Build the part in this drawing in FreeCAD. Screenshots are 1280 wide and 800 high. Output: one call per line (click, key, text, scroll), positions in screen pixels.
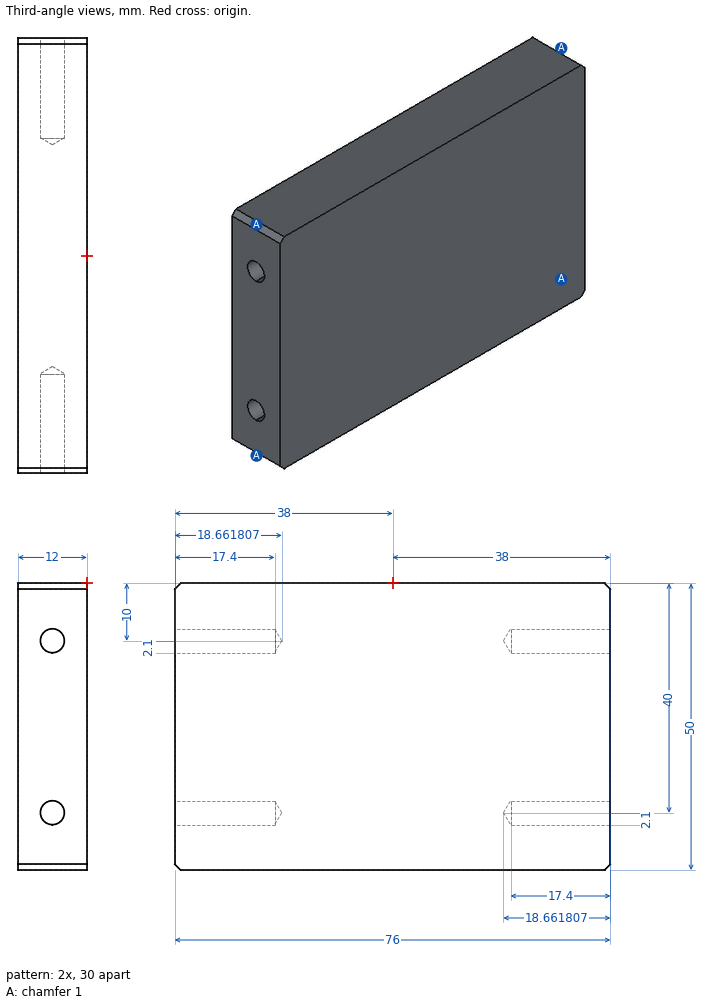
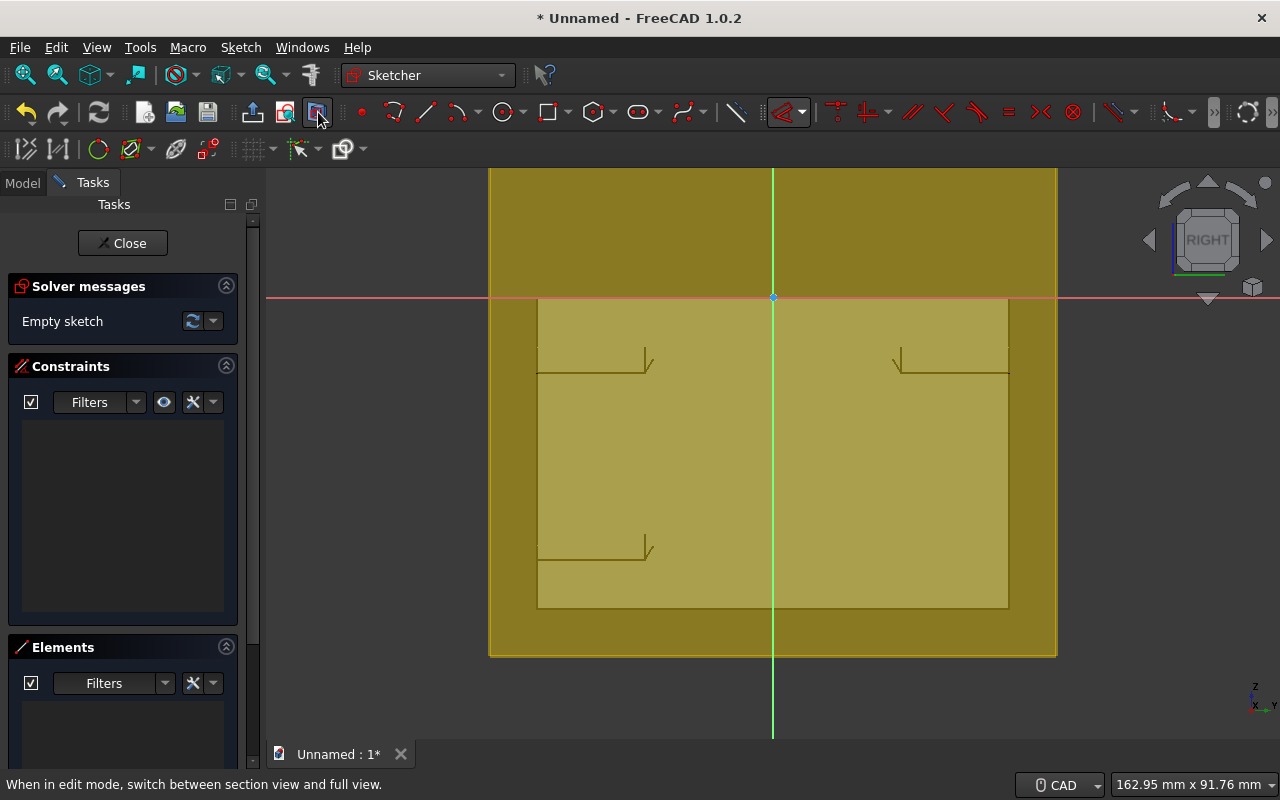
scroll(1115, 379, up, 2)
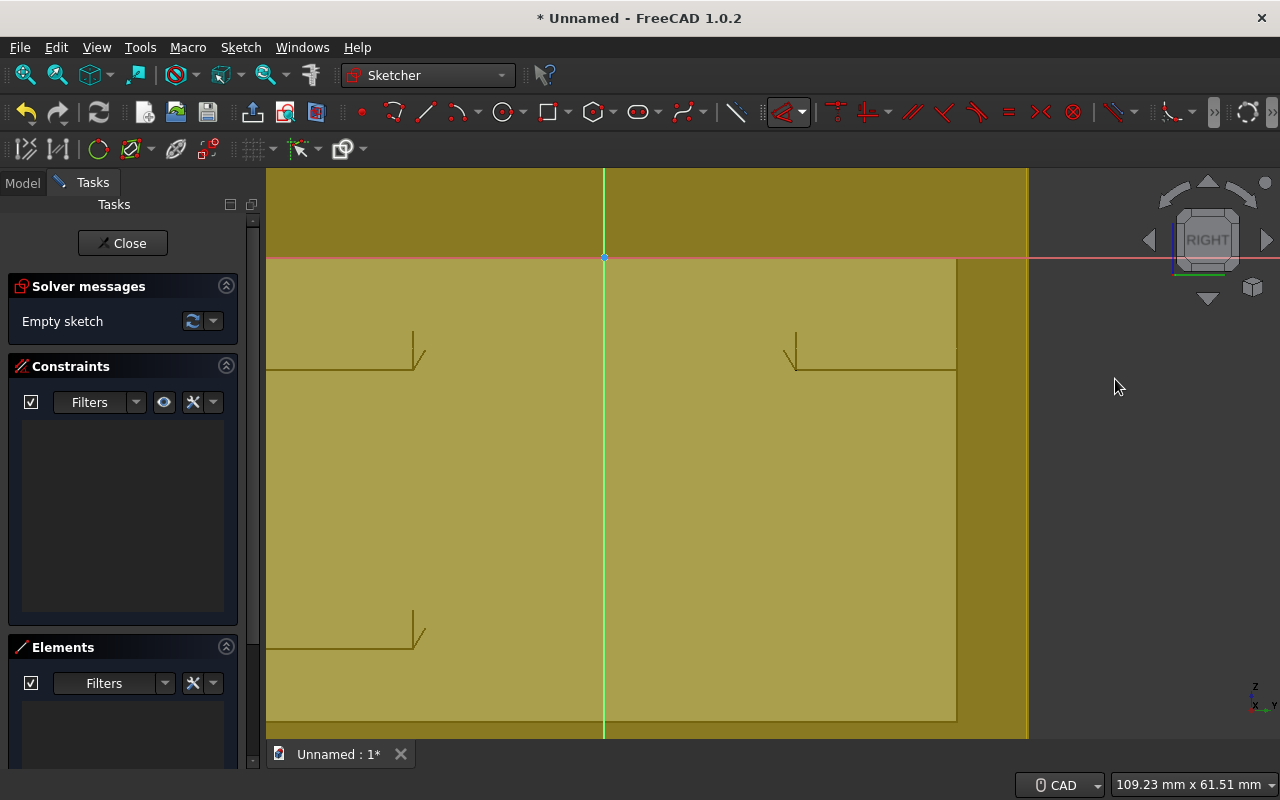
click(394, 112)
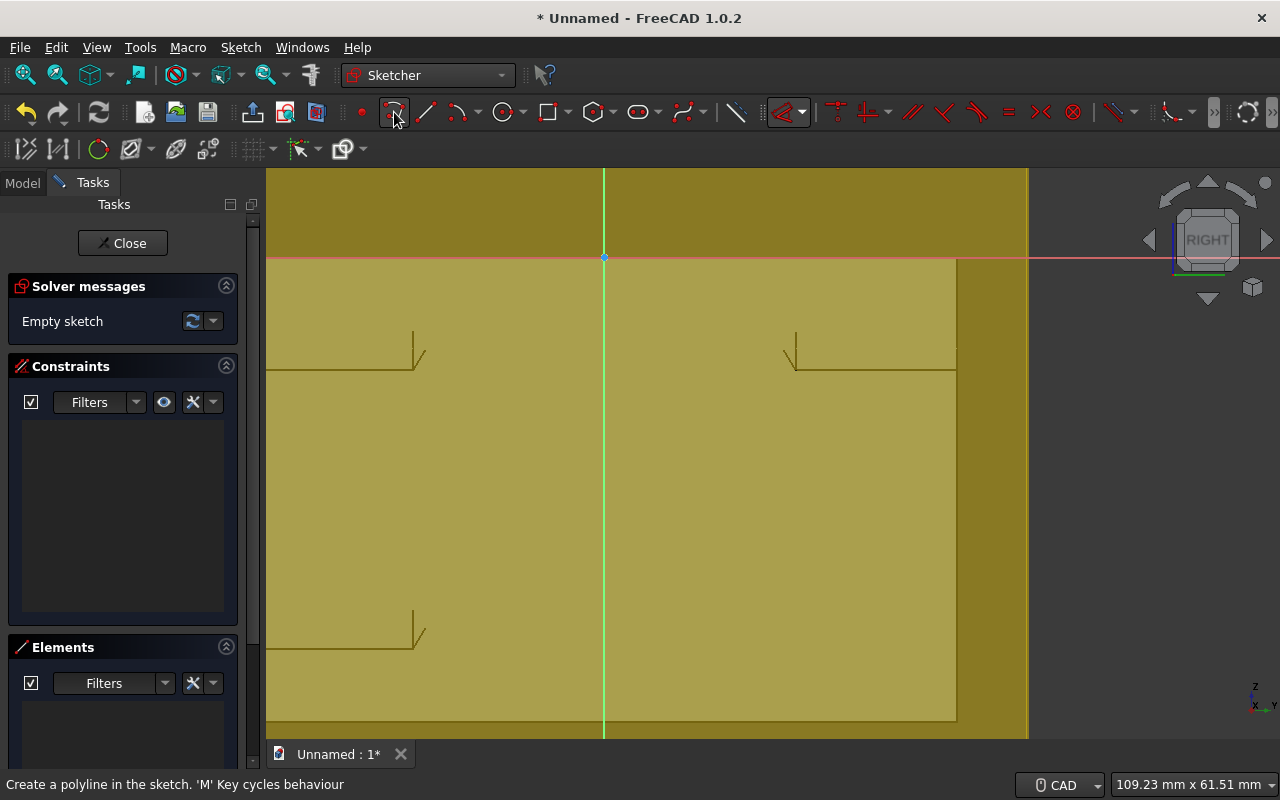
click(784, 629)
click(796, 649)
click(957, 649)
click(957, 629)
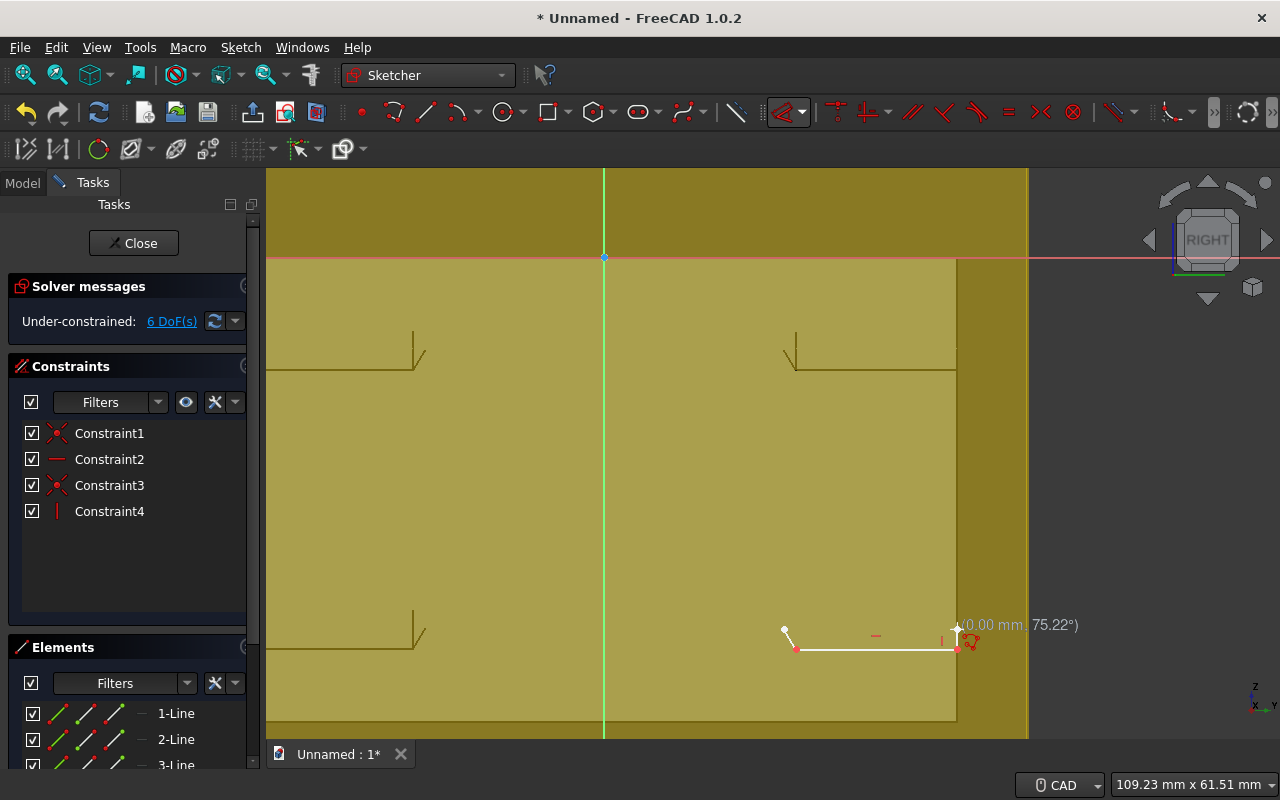
scroll(784, 629, up, 2)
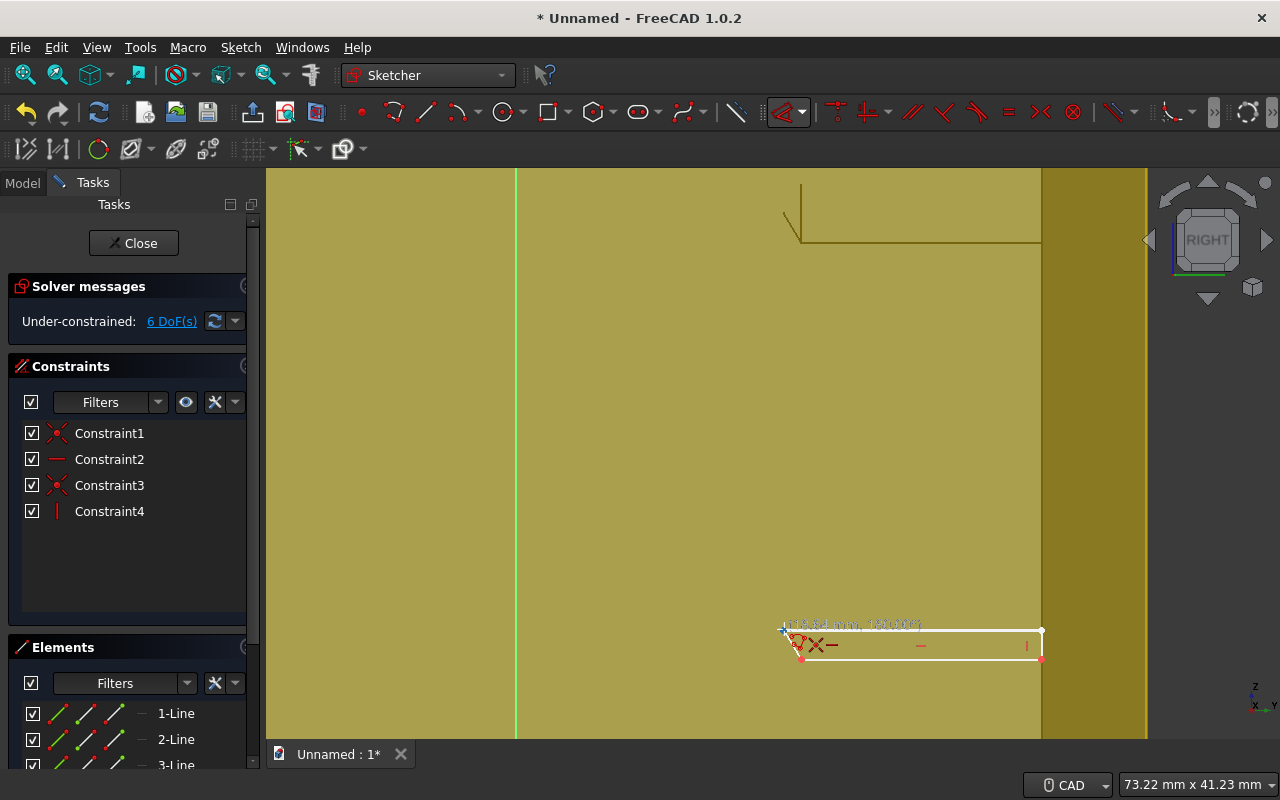
click(784, 630)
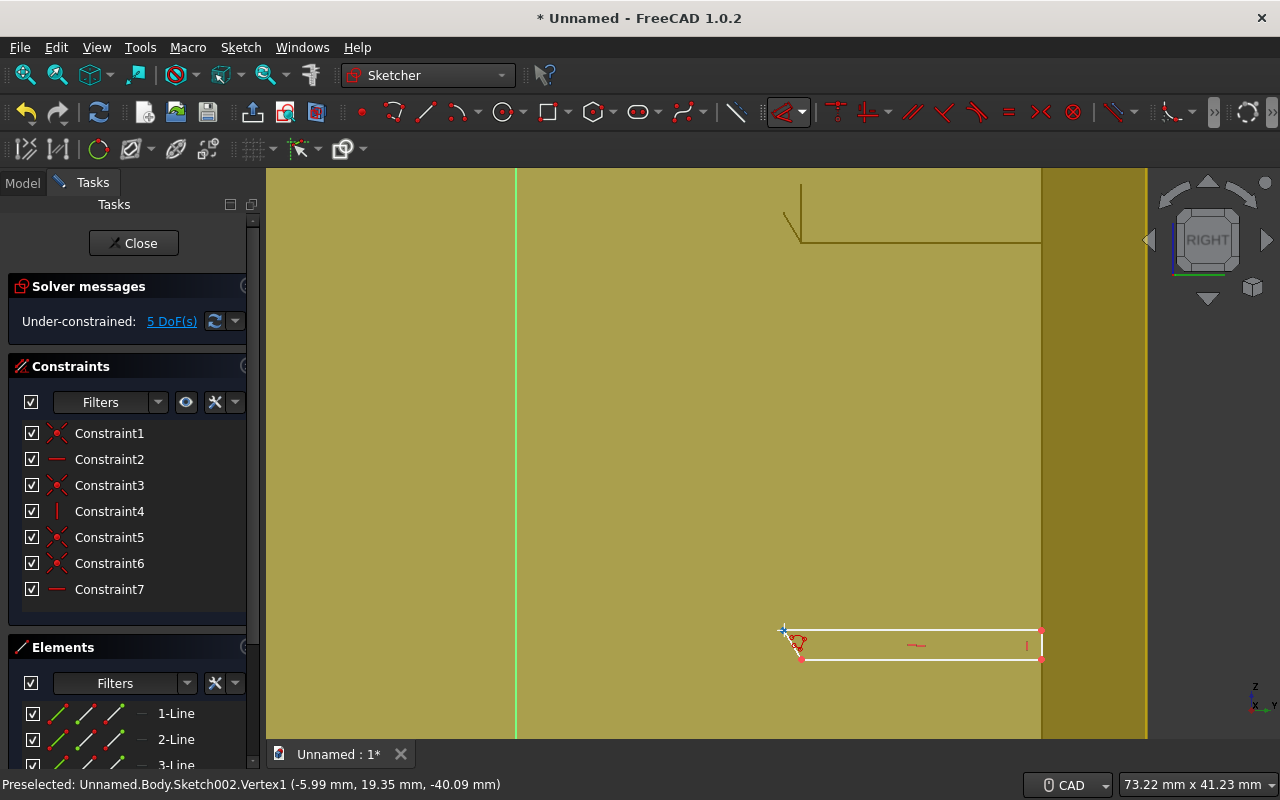
click(426, 112)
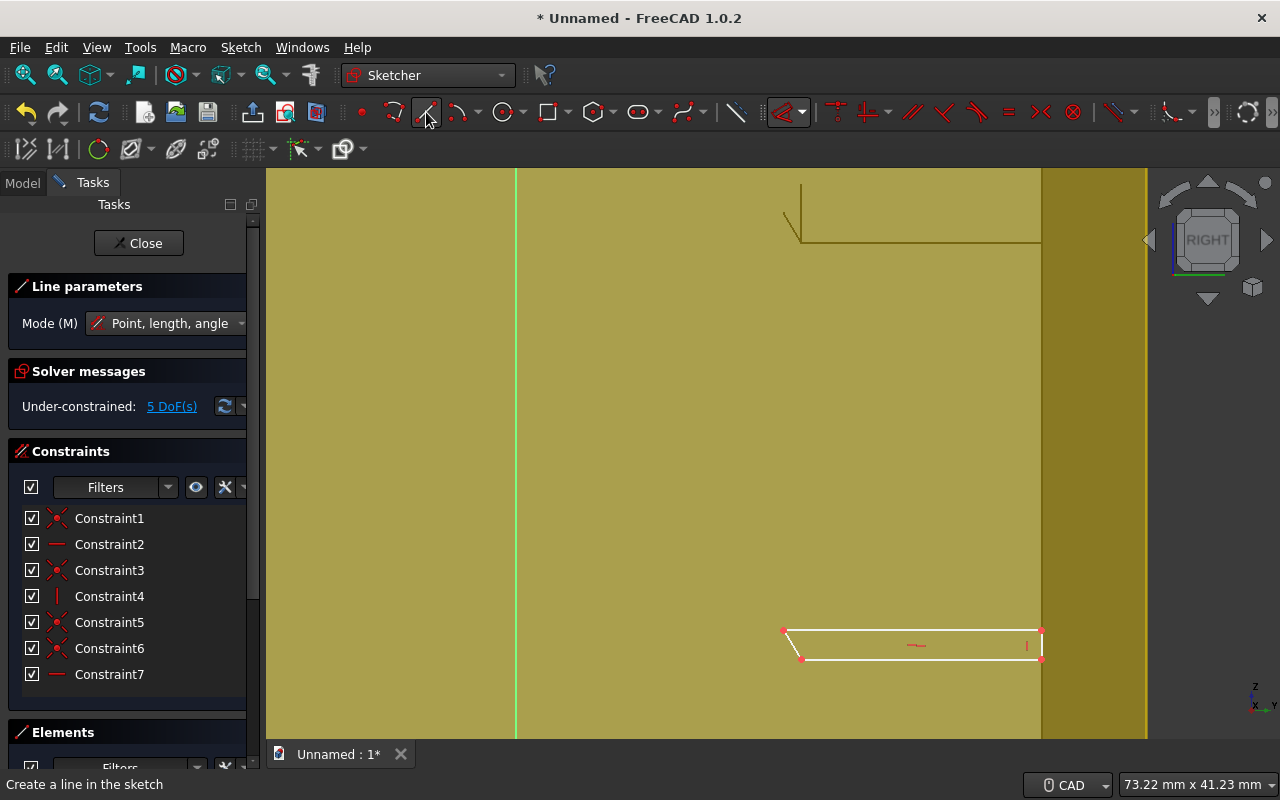
click(1068, 629)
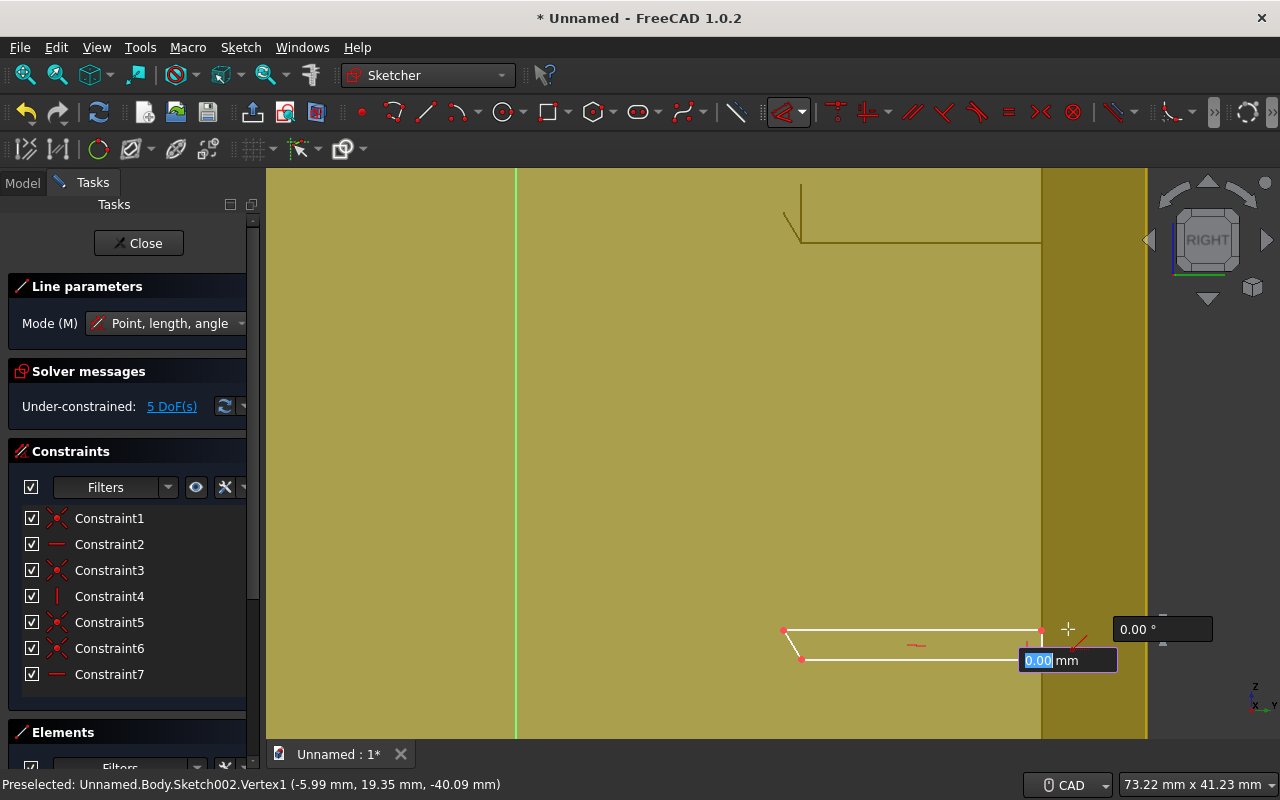
scroll(448, 630, down, 2)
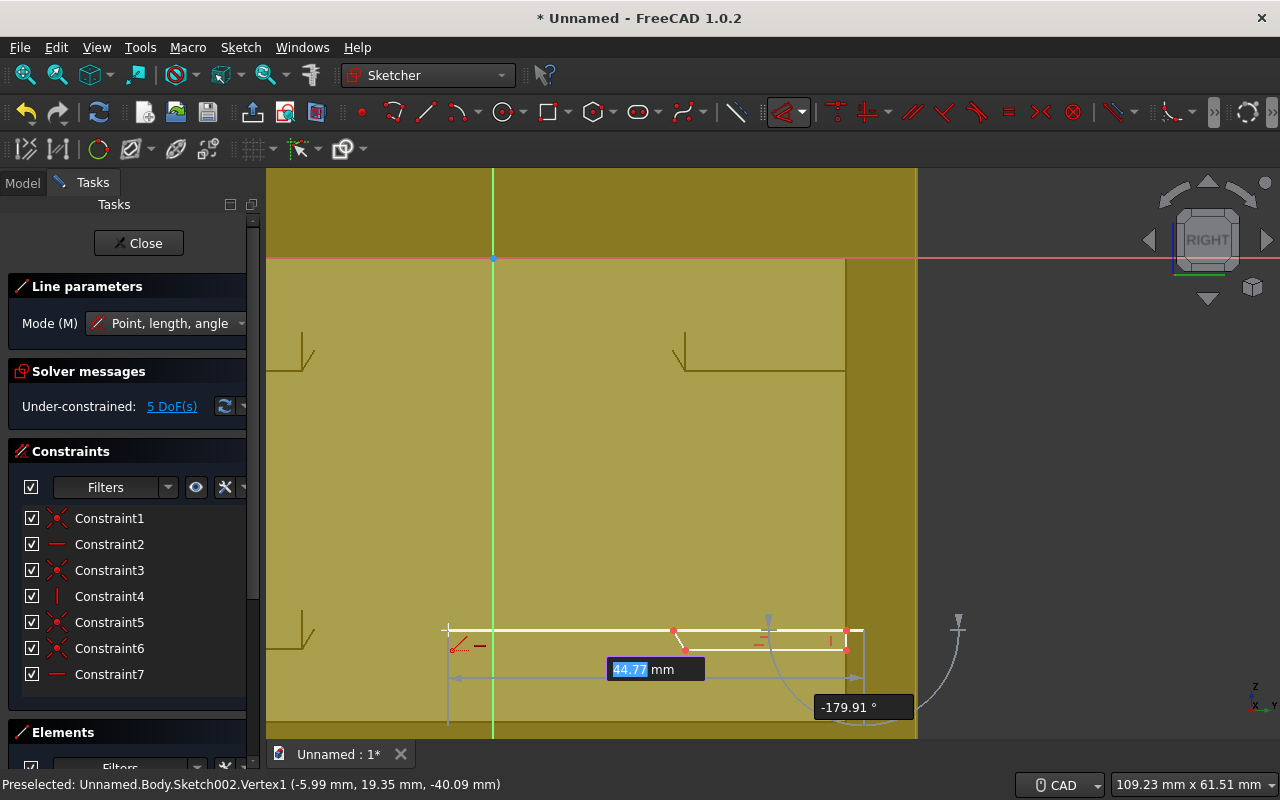
click(916, 630)
key(Escape)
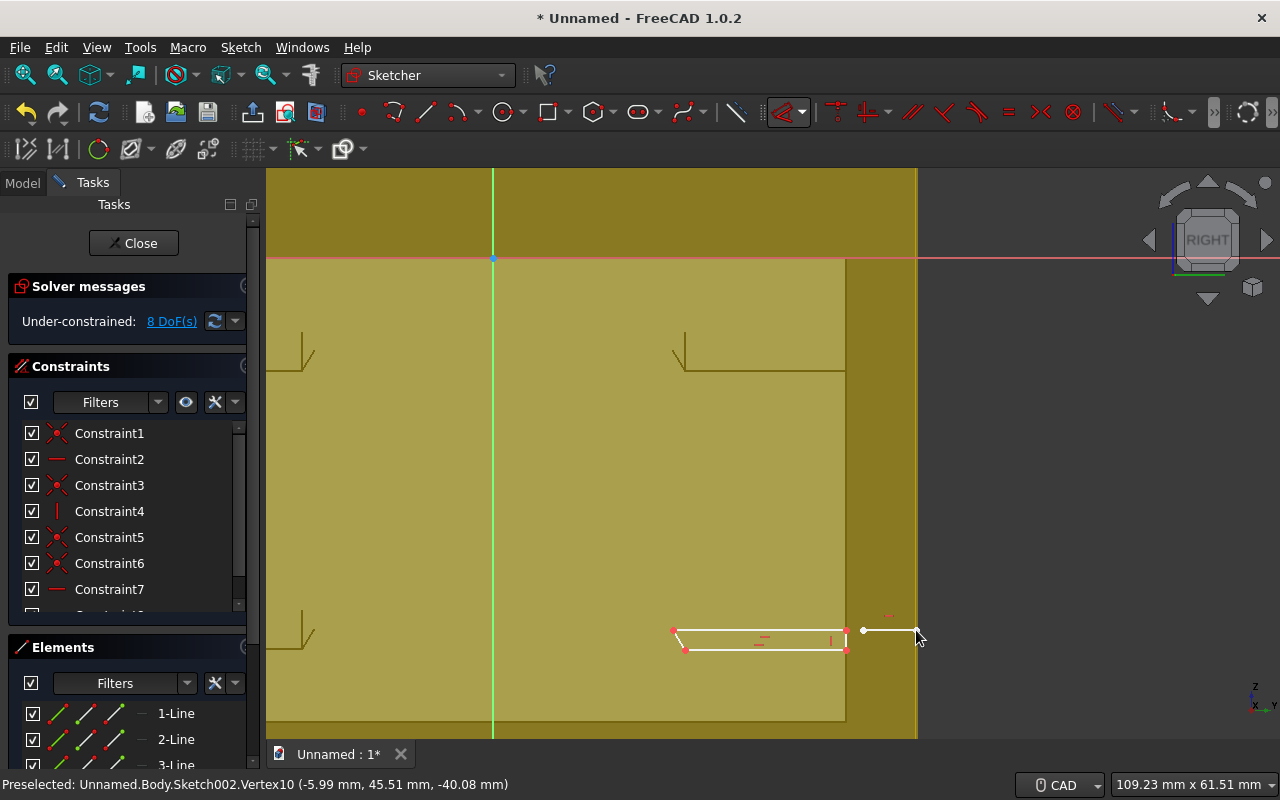
click(879, 630)